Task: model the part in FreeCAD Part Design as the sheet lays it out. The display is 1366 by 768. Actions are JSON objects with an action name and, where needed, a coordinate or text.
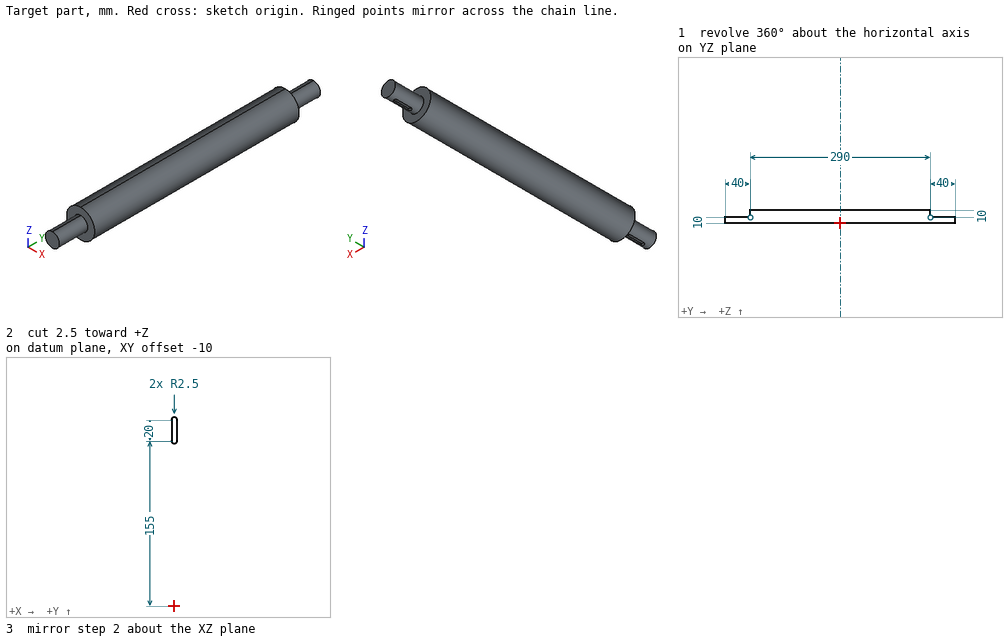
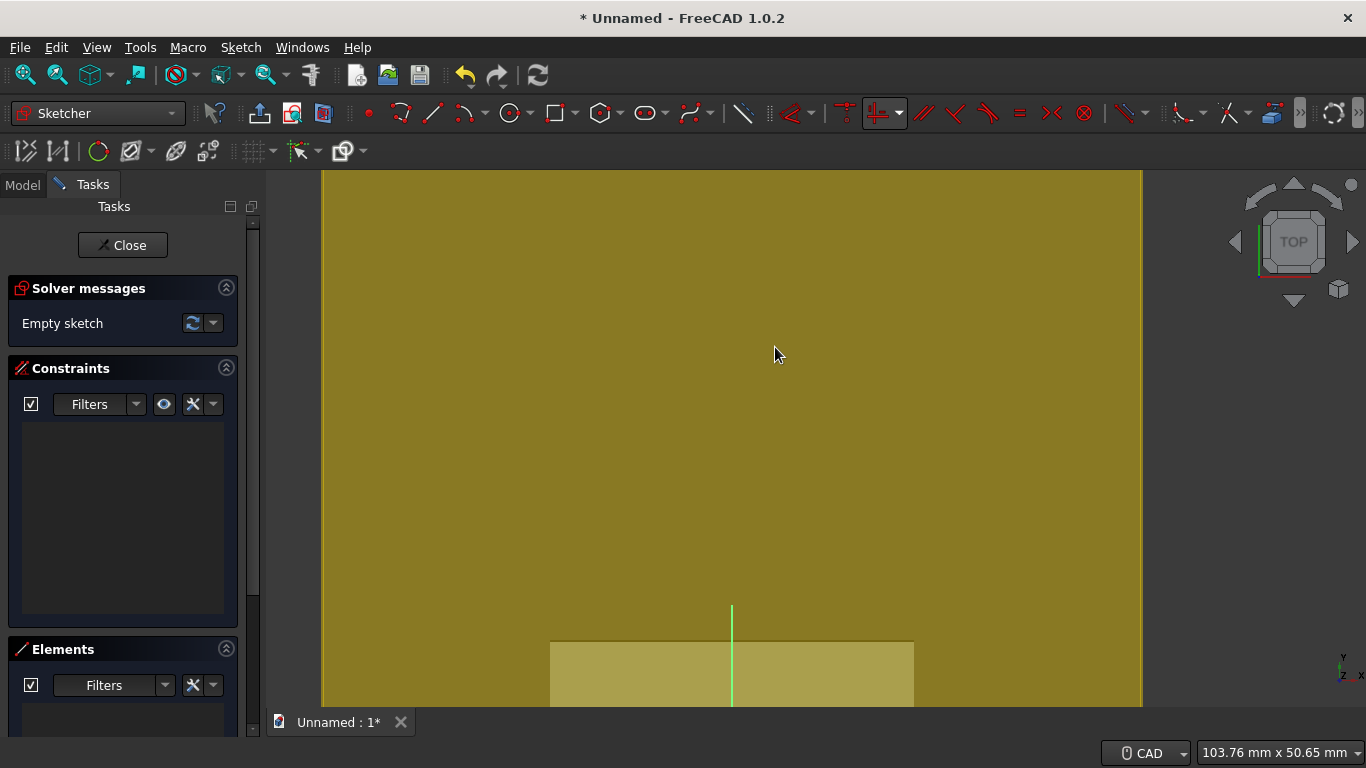
{"action": "left_click", "coordinate": [732, 535]}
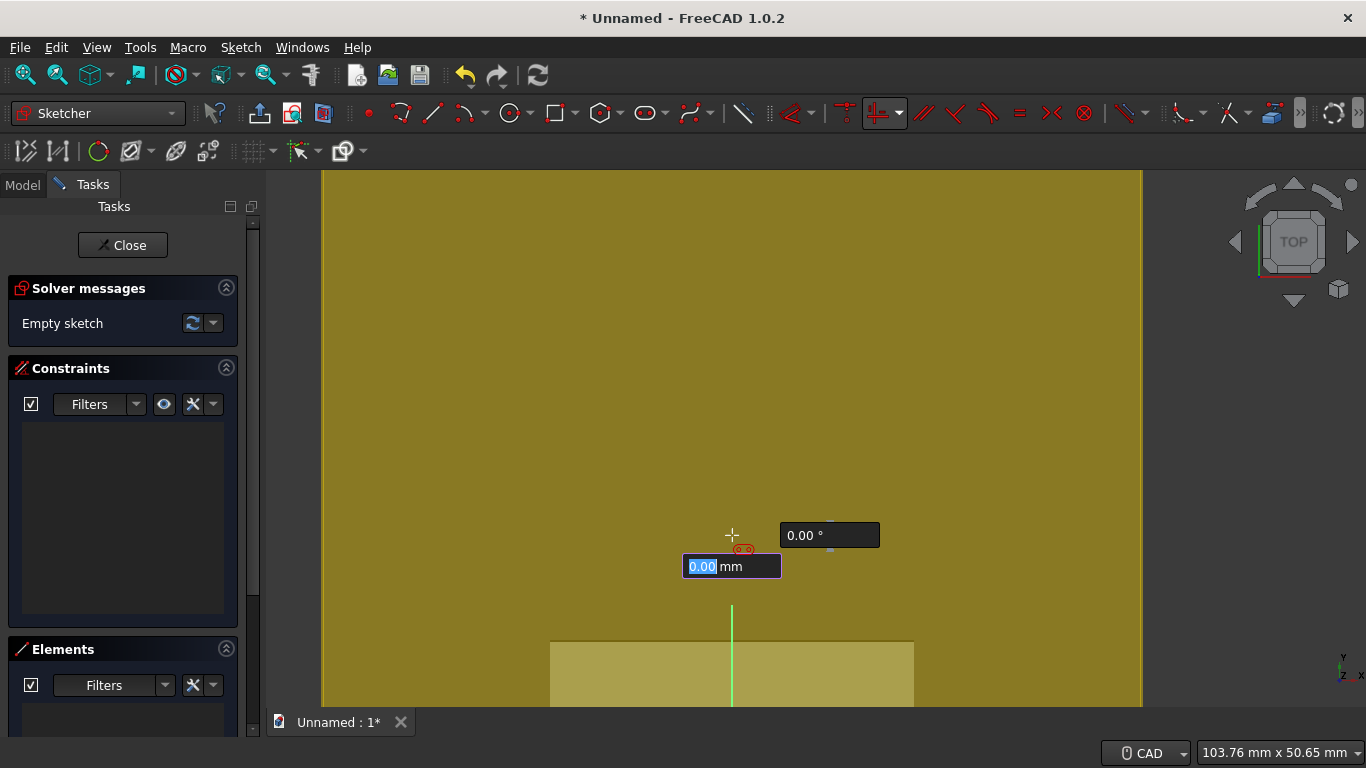
{"action": "left_click", "coordinate": [741, 323]}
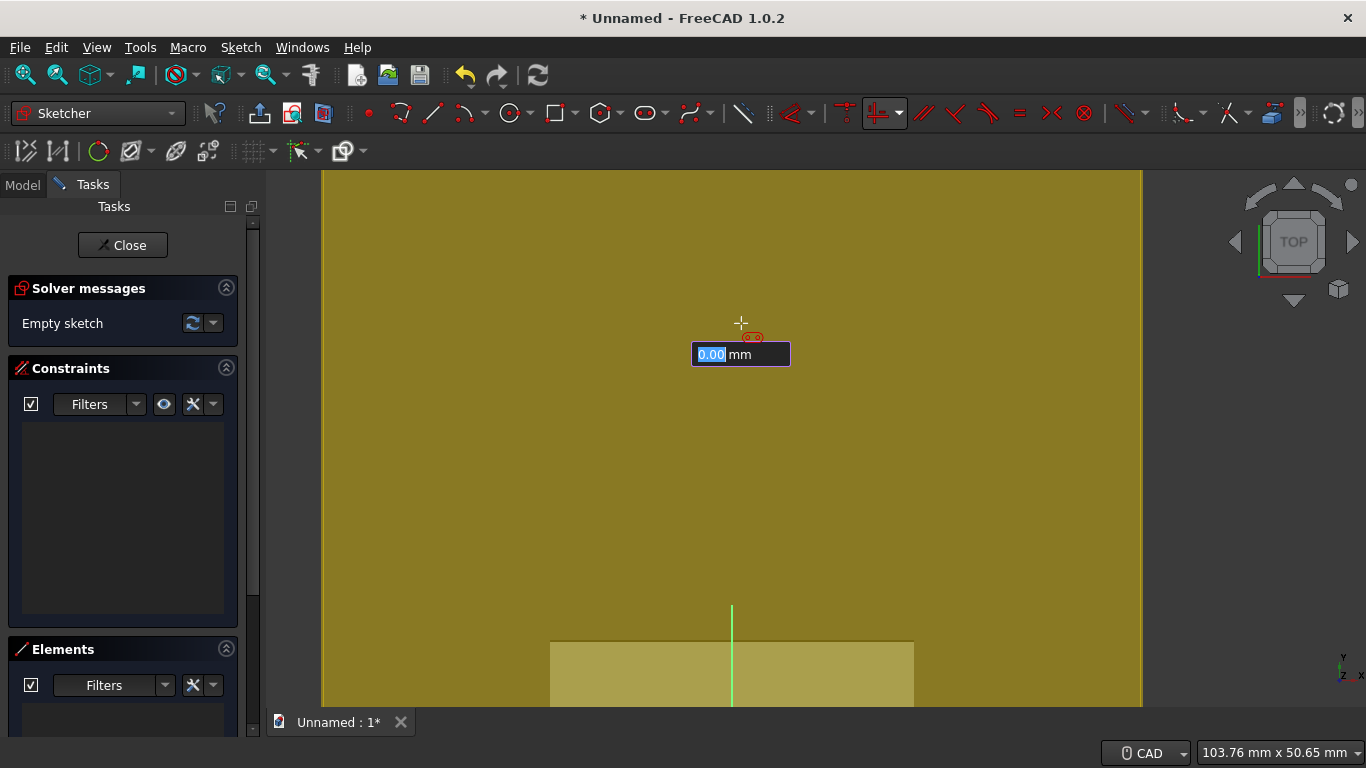
{"action": "left_click", "coordinate": [705, 429]}
{"action": "key", "text": "Escape"}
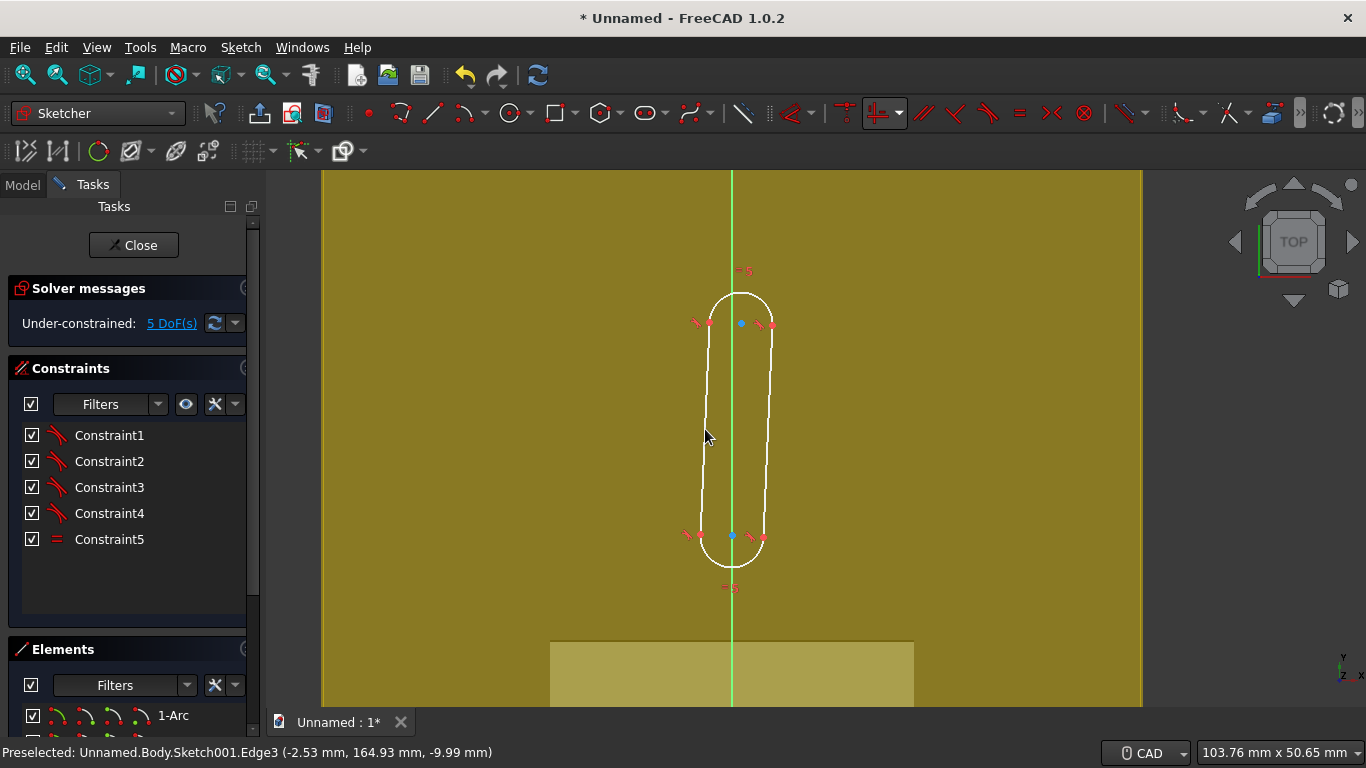
{"action": "left_click", "coordinate": [703, 471]}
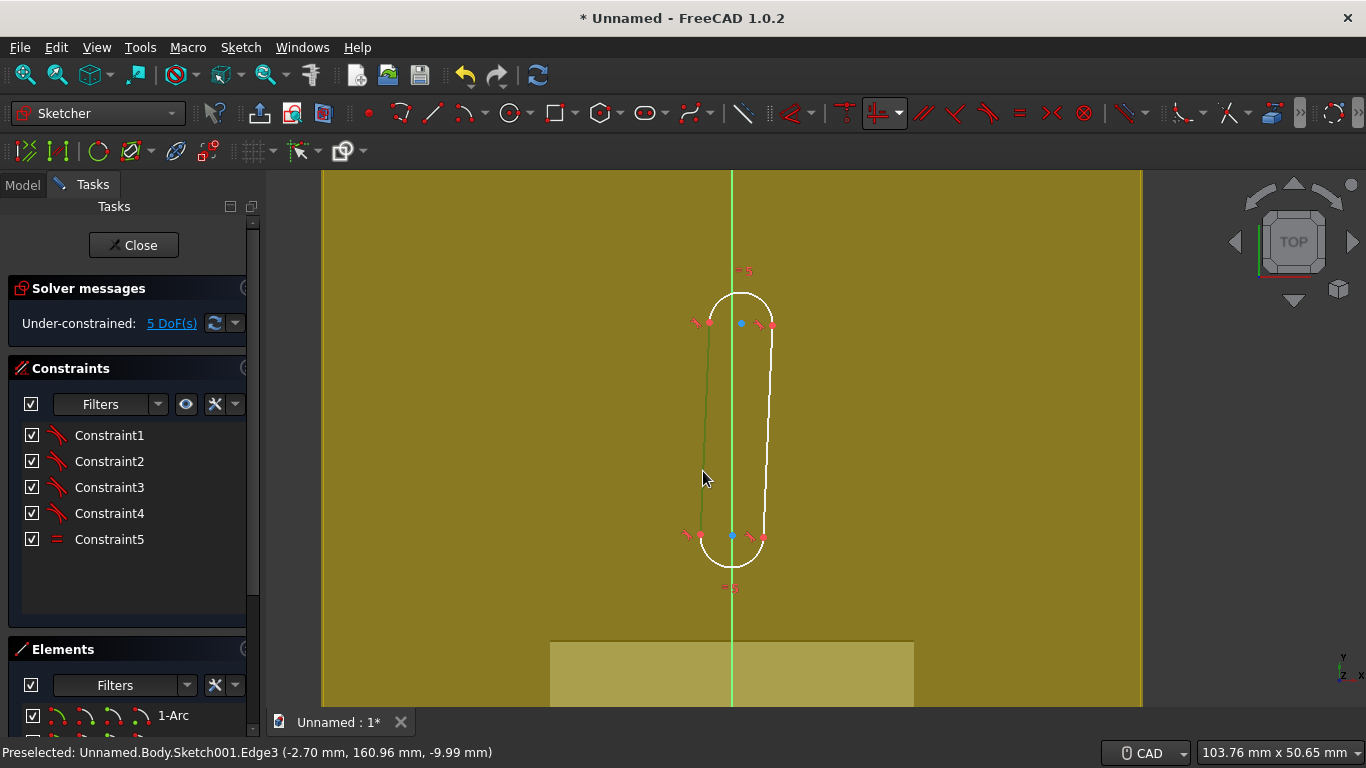
{"action": "key", "text": "v"}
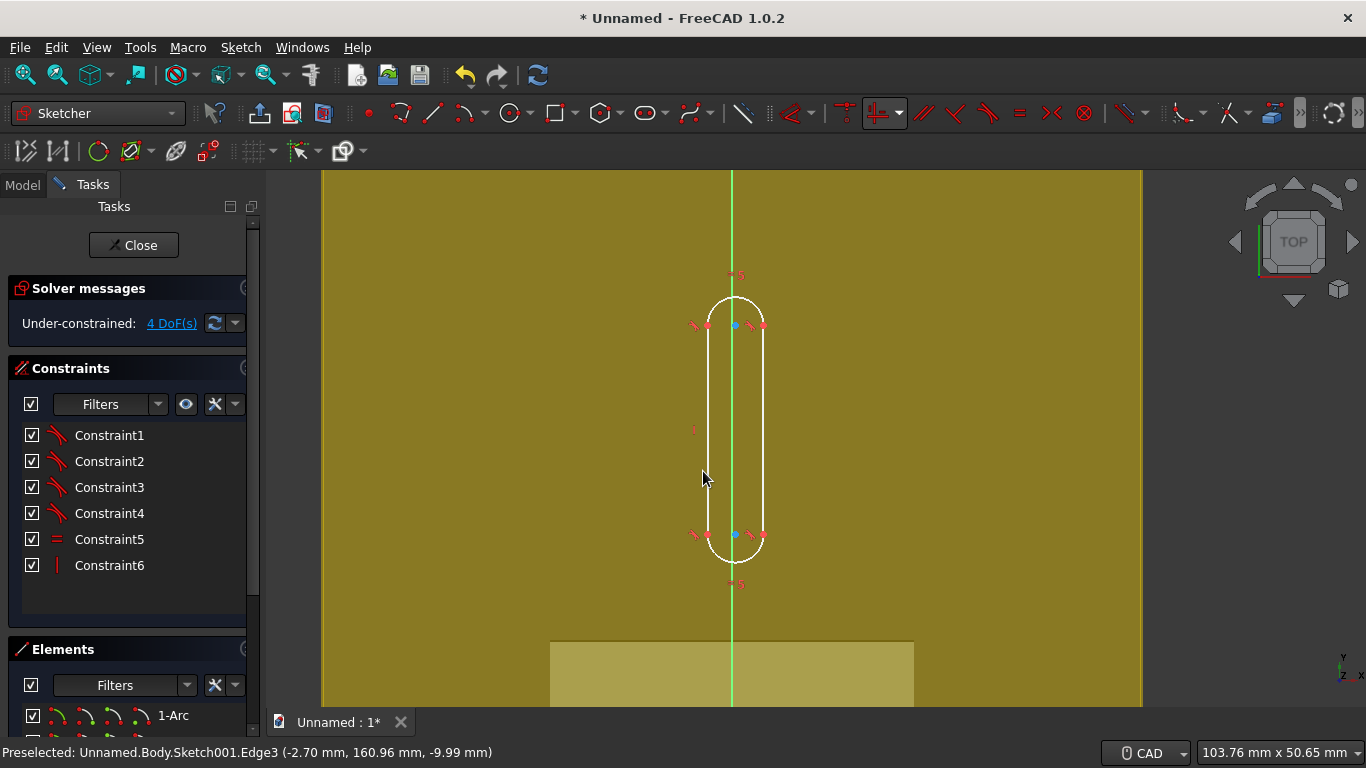
{"action": "left_click", "coordinate": [736, 535]}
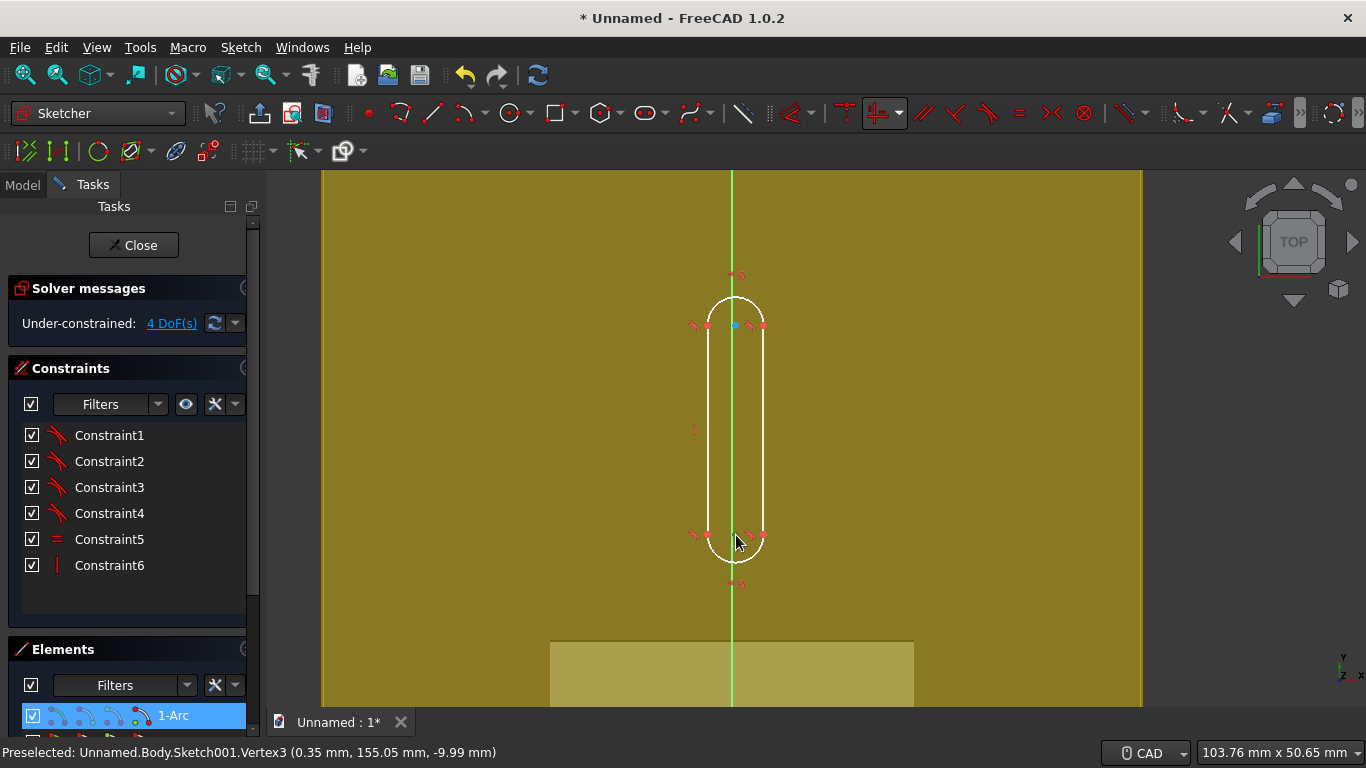
{"action": "left_click", "coordinate": [732, 645]}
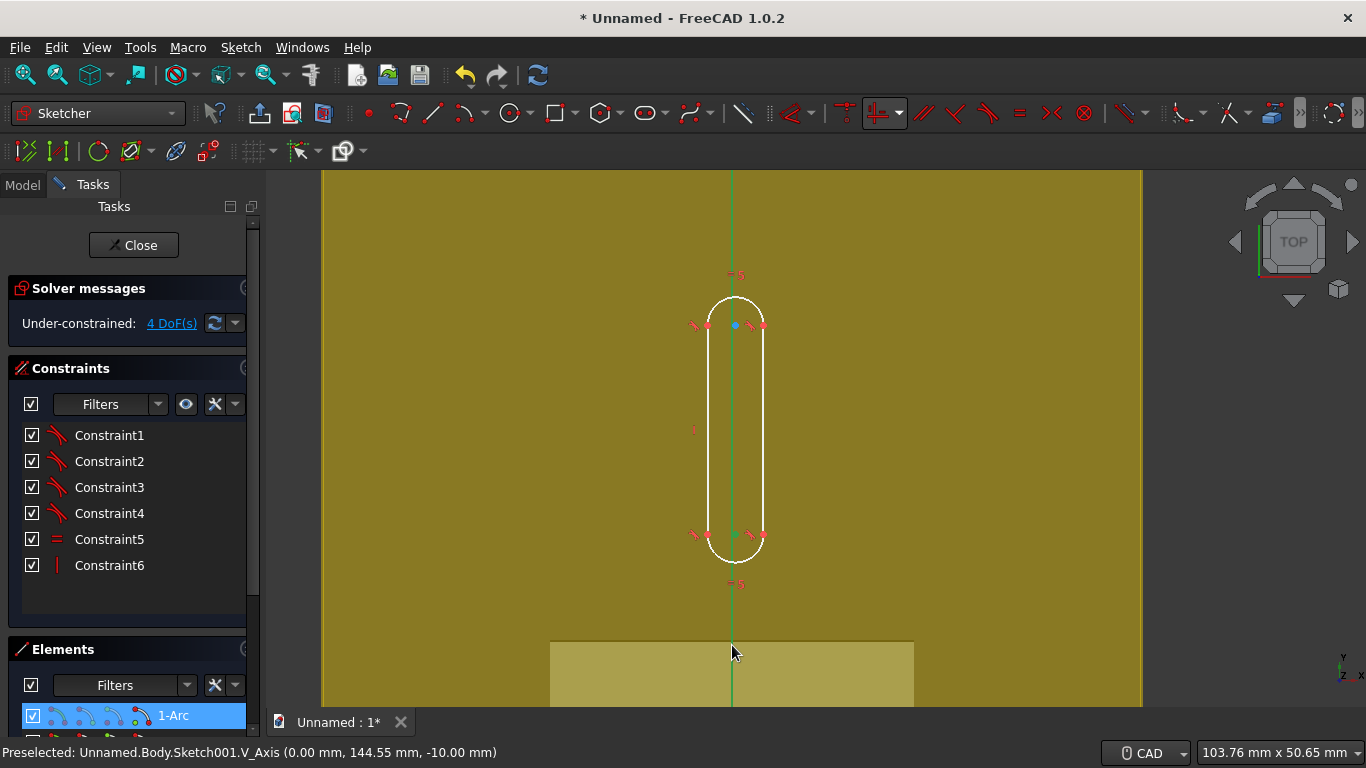
{"action": "key", "text": "c"}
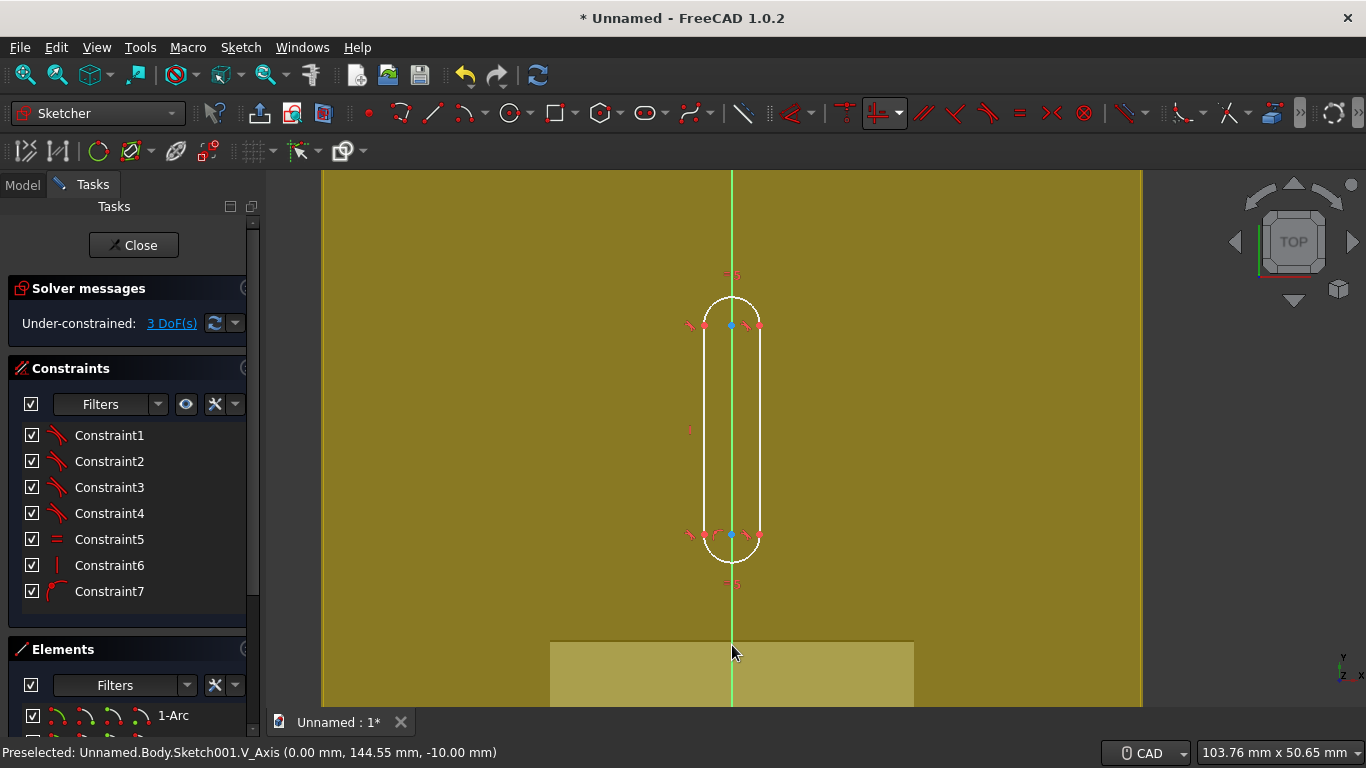
{"action": "key", "text": "d"}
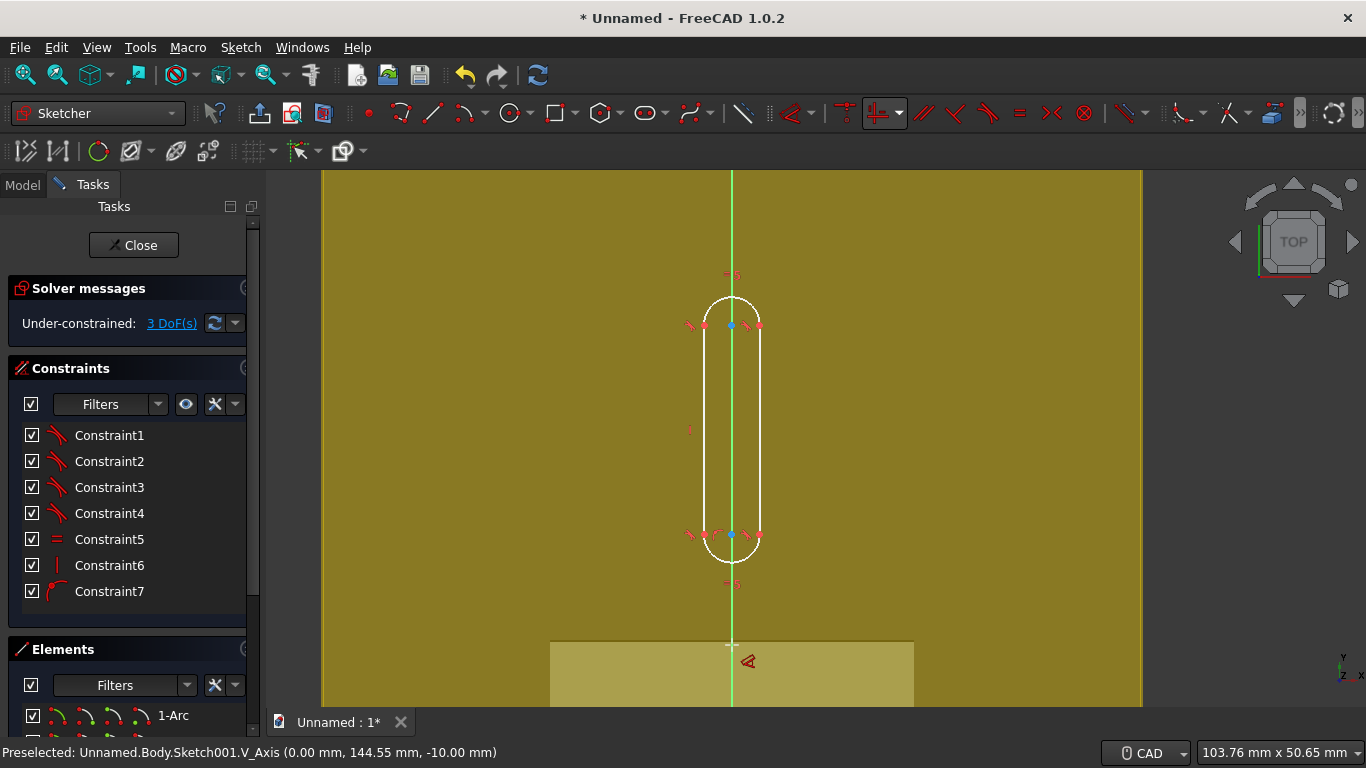
{"action": "scroll", "coordinate": [715, 557], "scroll_direction": "up", "scroll_amount": 3}